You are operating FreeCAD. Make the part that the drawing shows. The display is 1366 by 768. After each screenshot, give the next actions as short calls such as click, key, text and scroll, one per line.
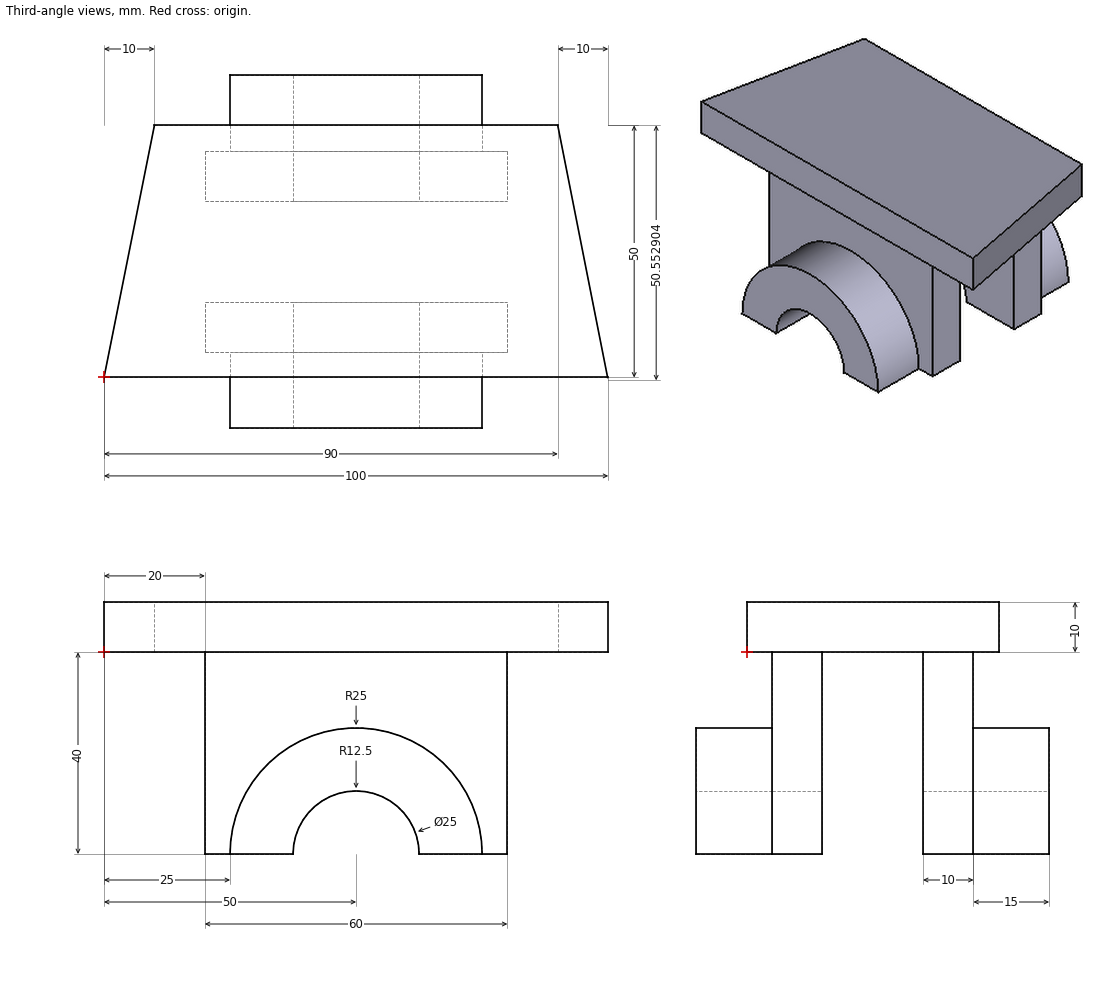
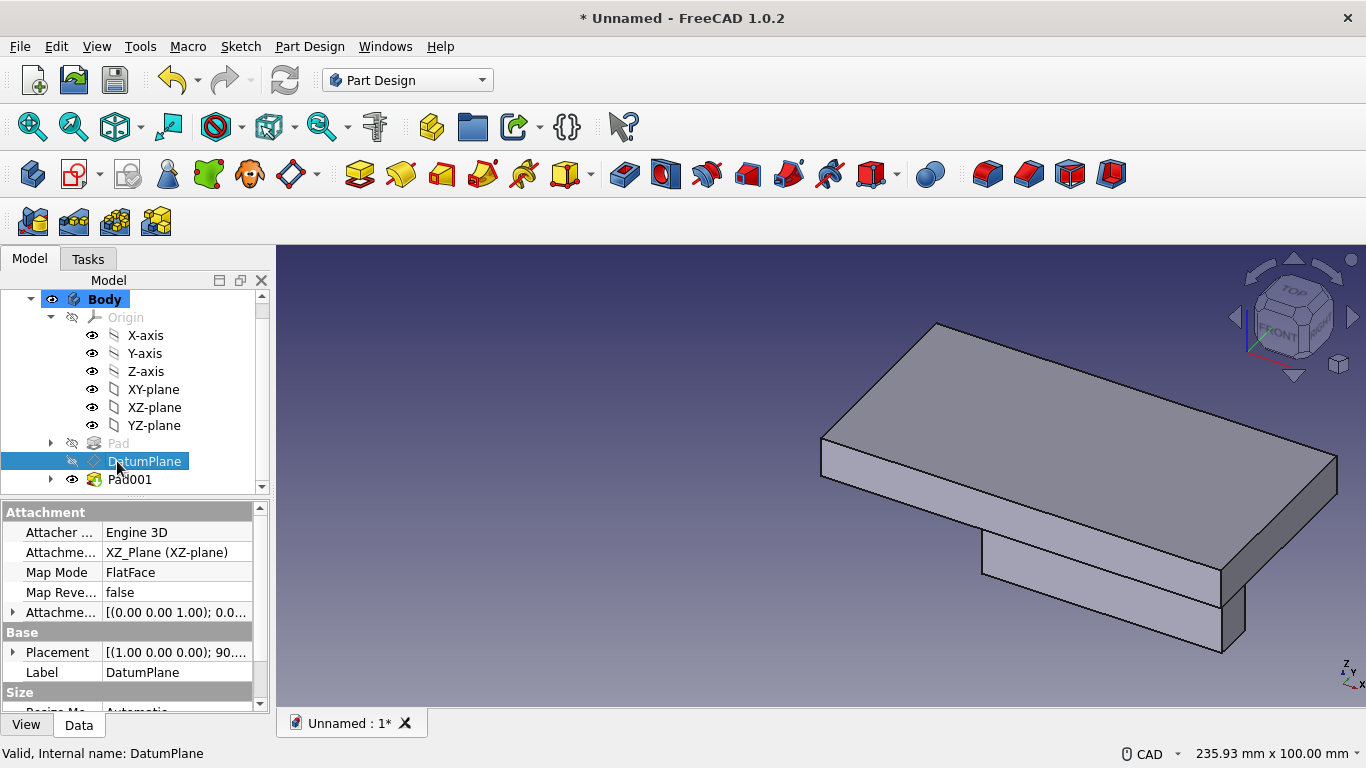
key(v)
key(f)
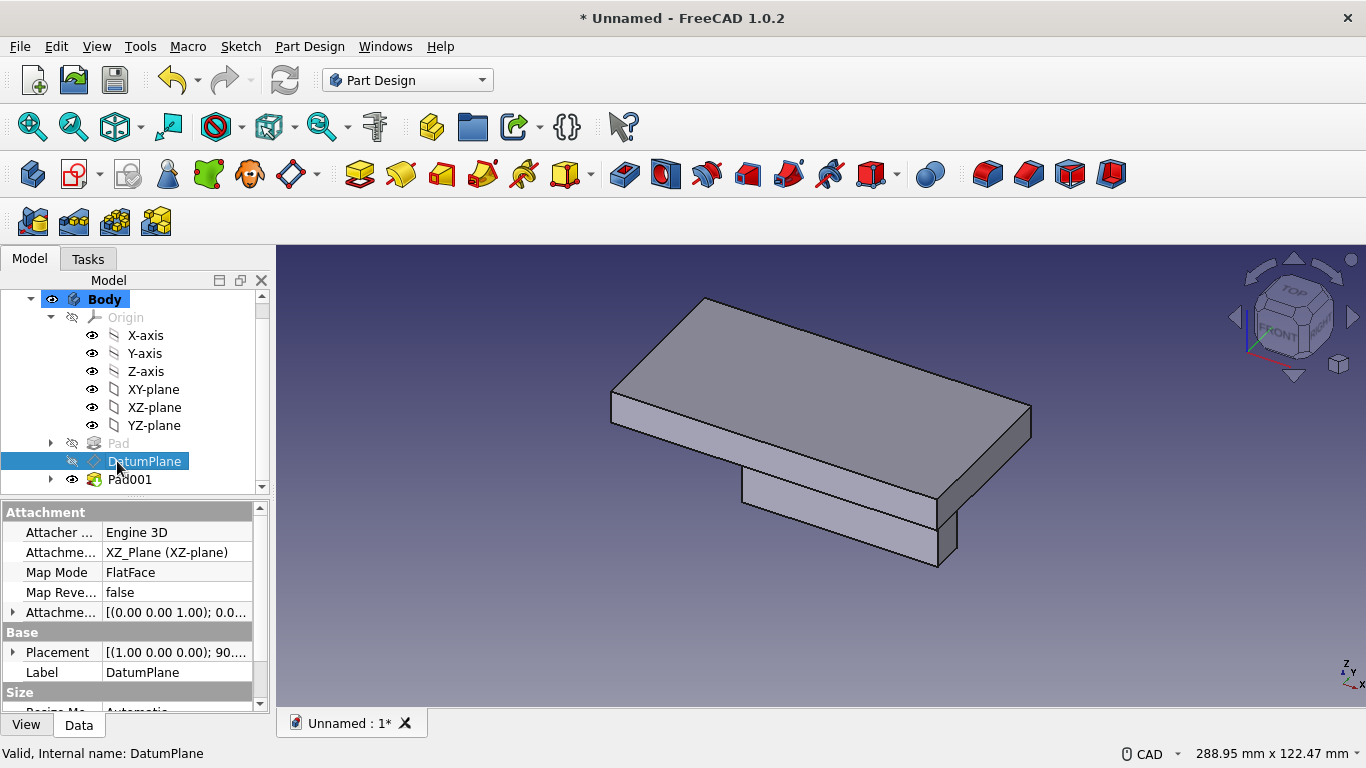
click(137, 407)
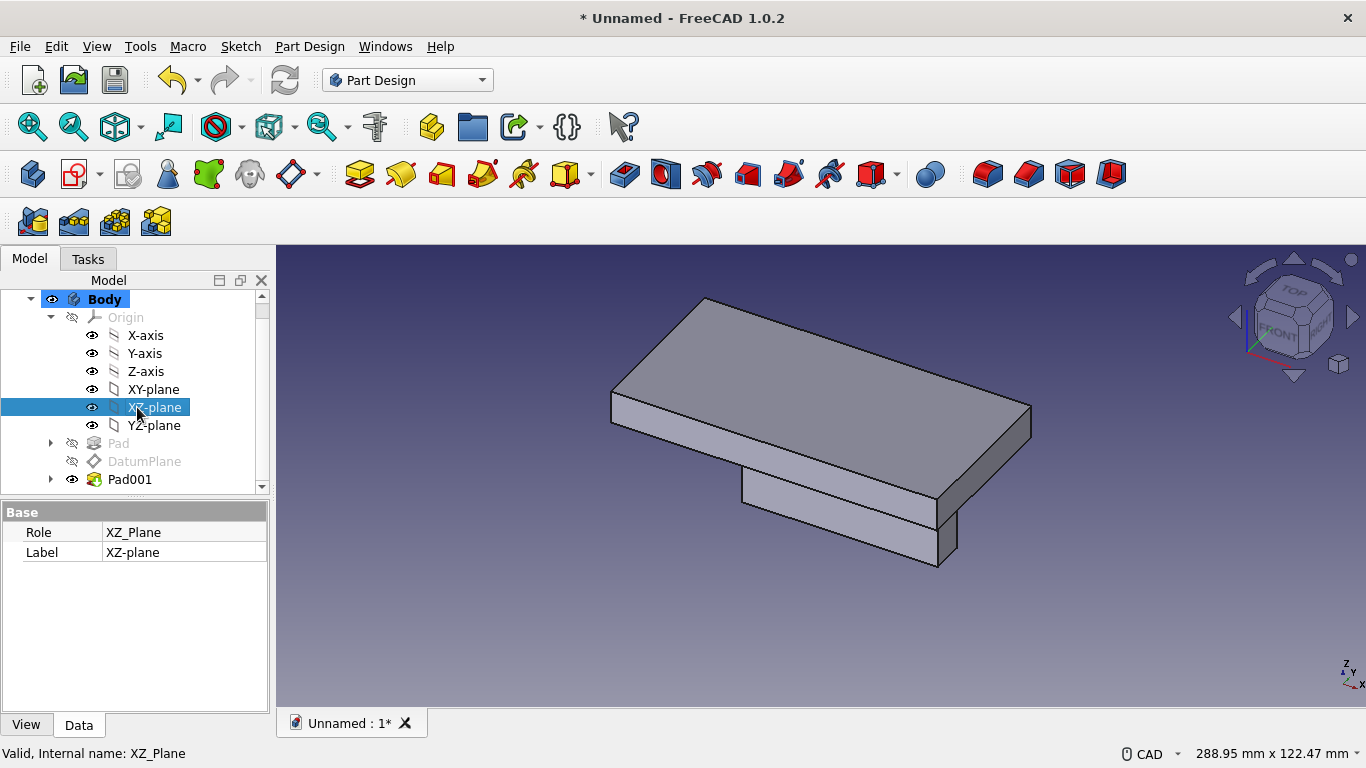
click(290, 174)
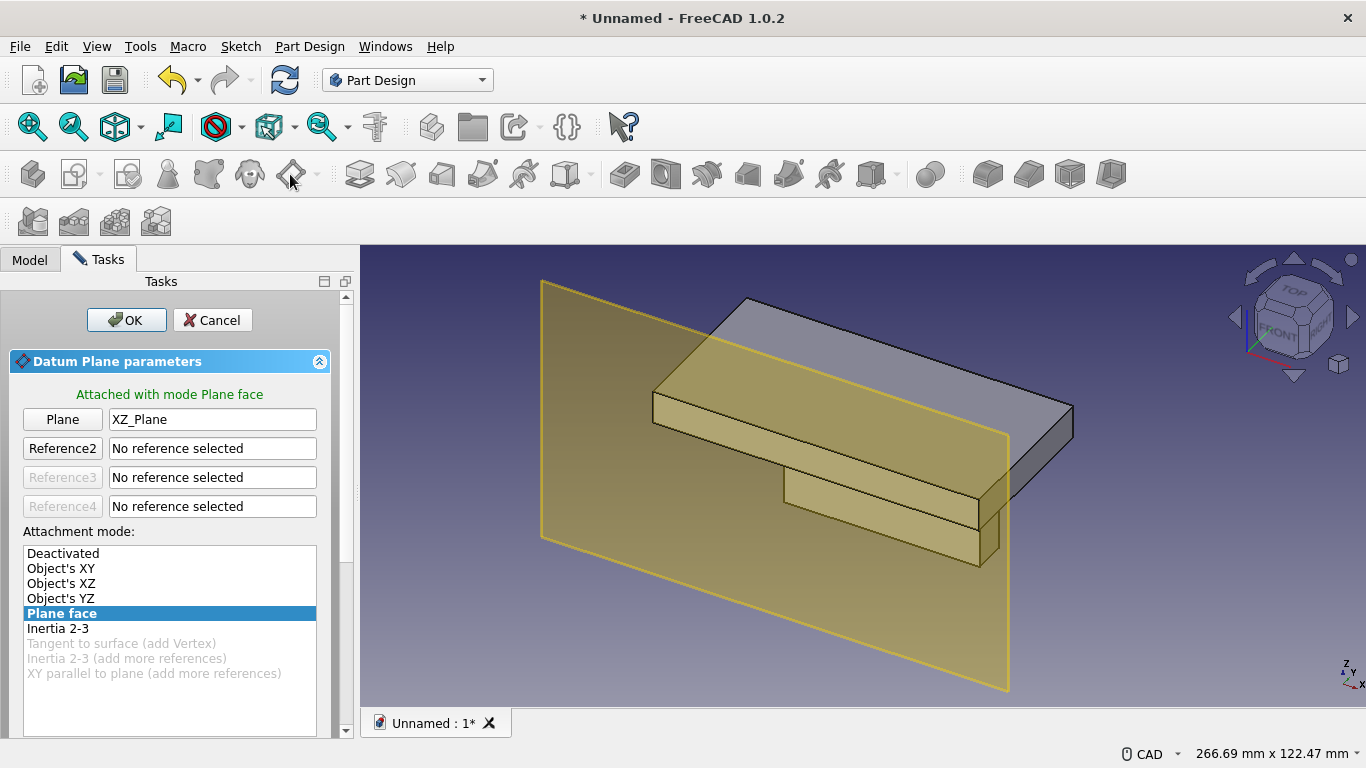
scroll(346, 514, down, 4)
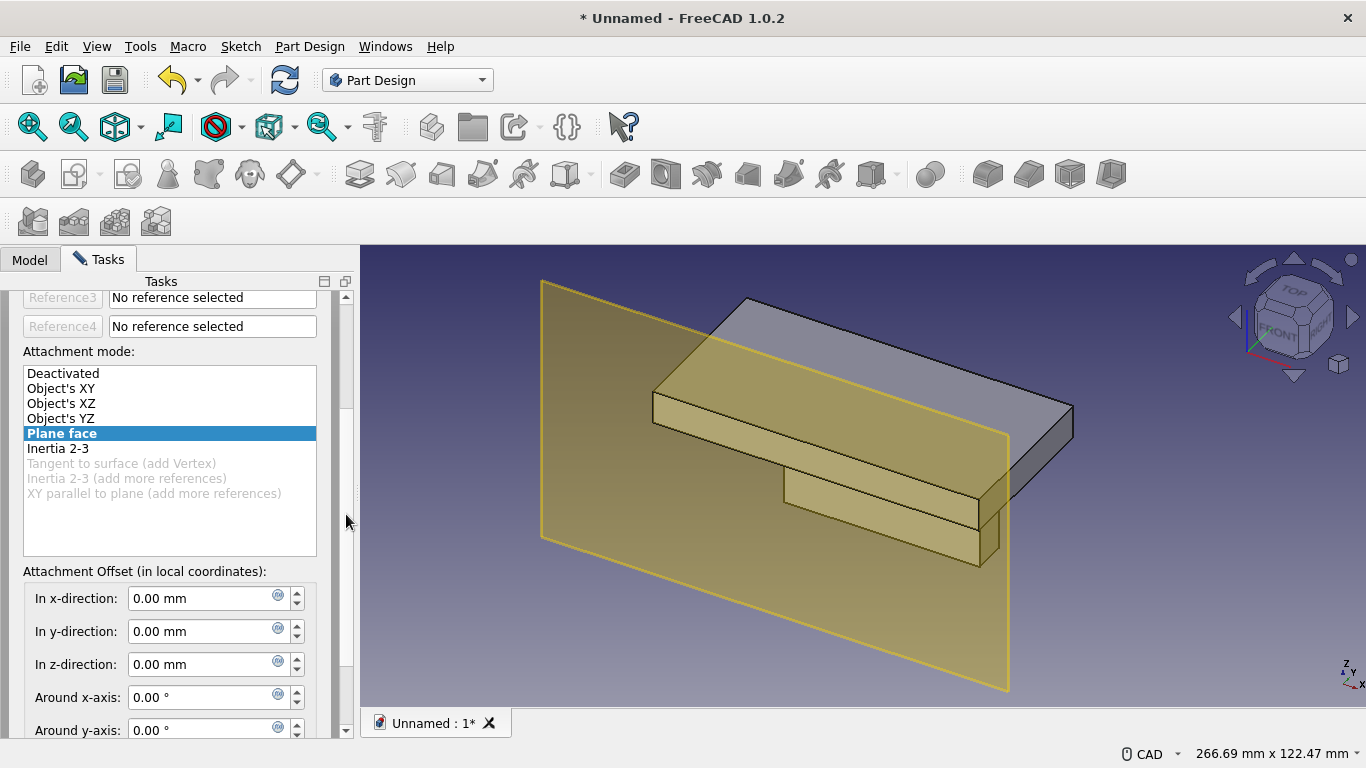
triple_click(210, 604)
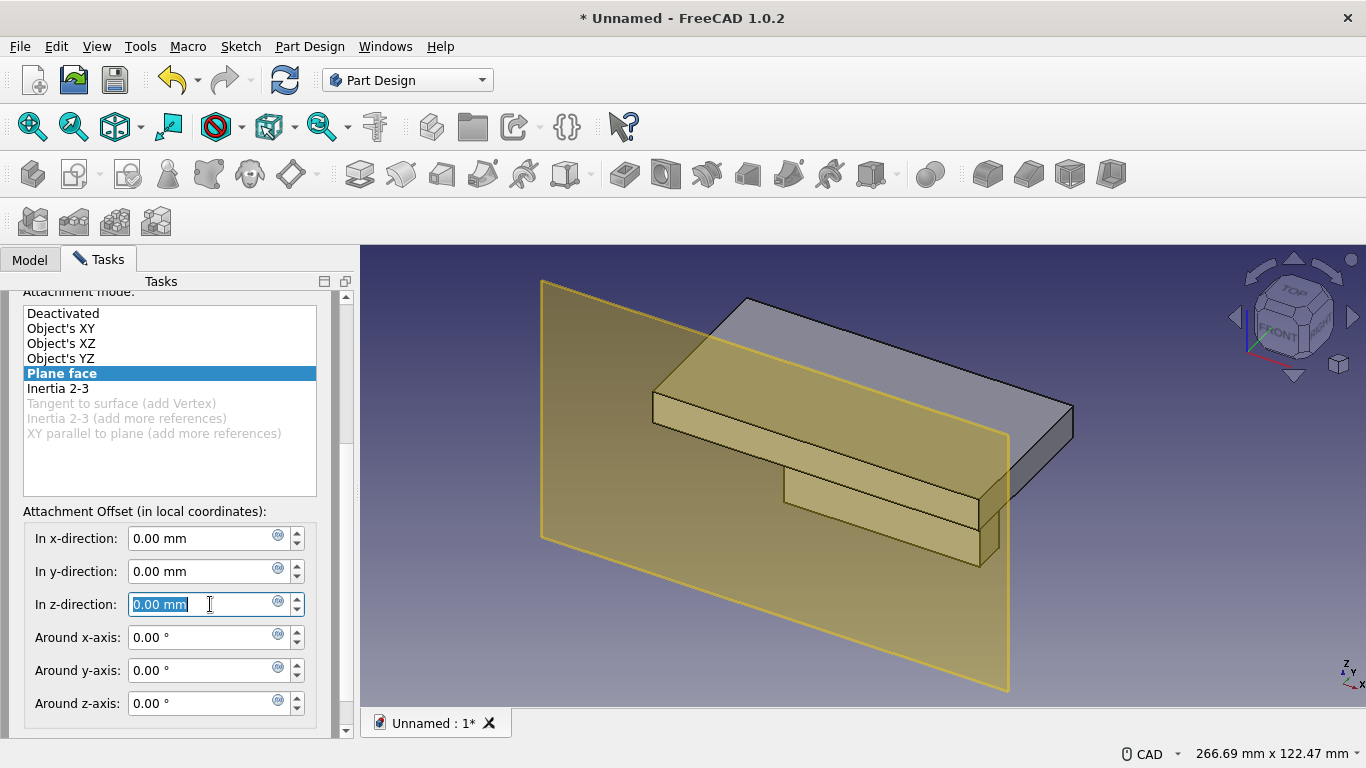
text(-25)
key(Tab)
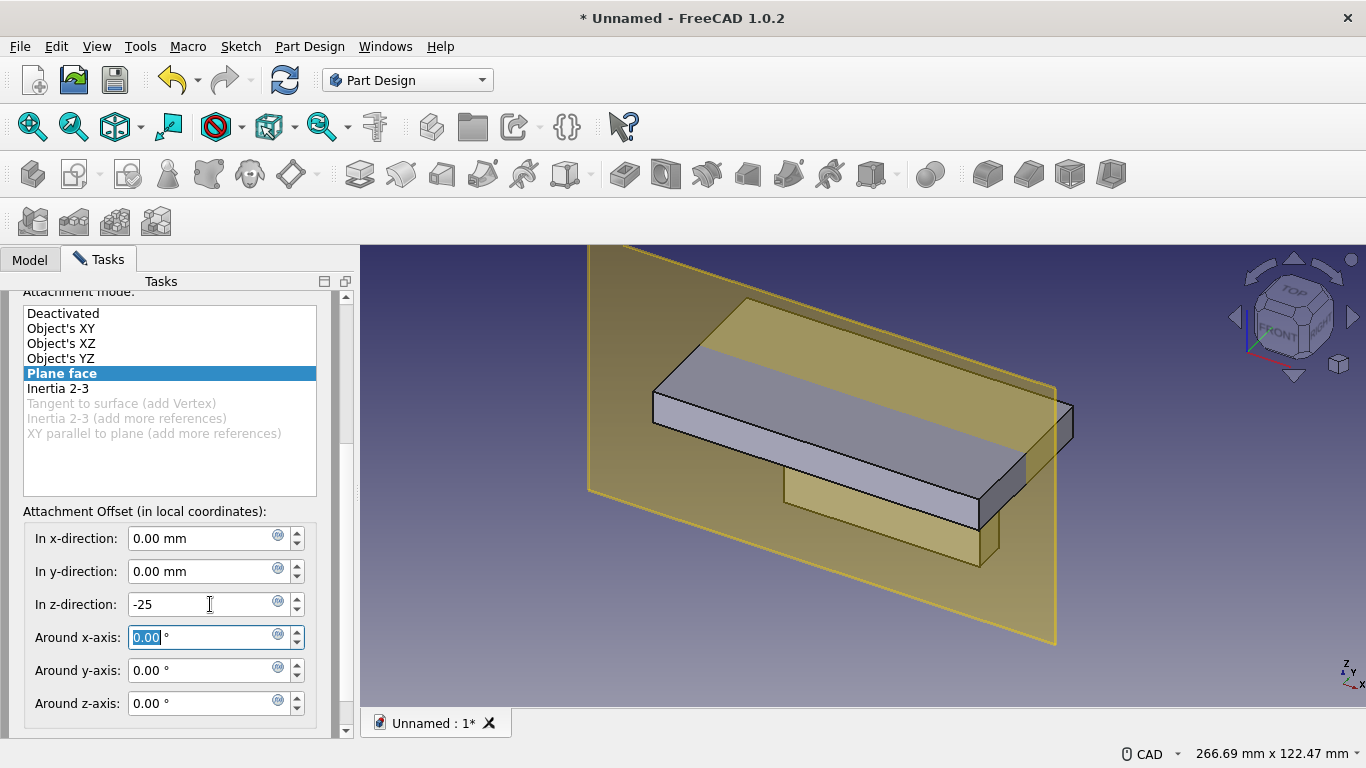
scroll(346, 514, up, 5)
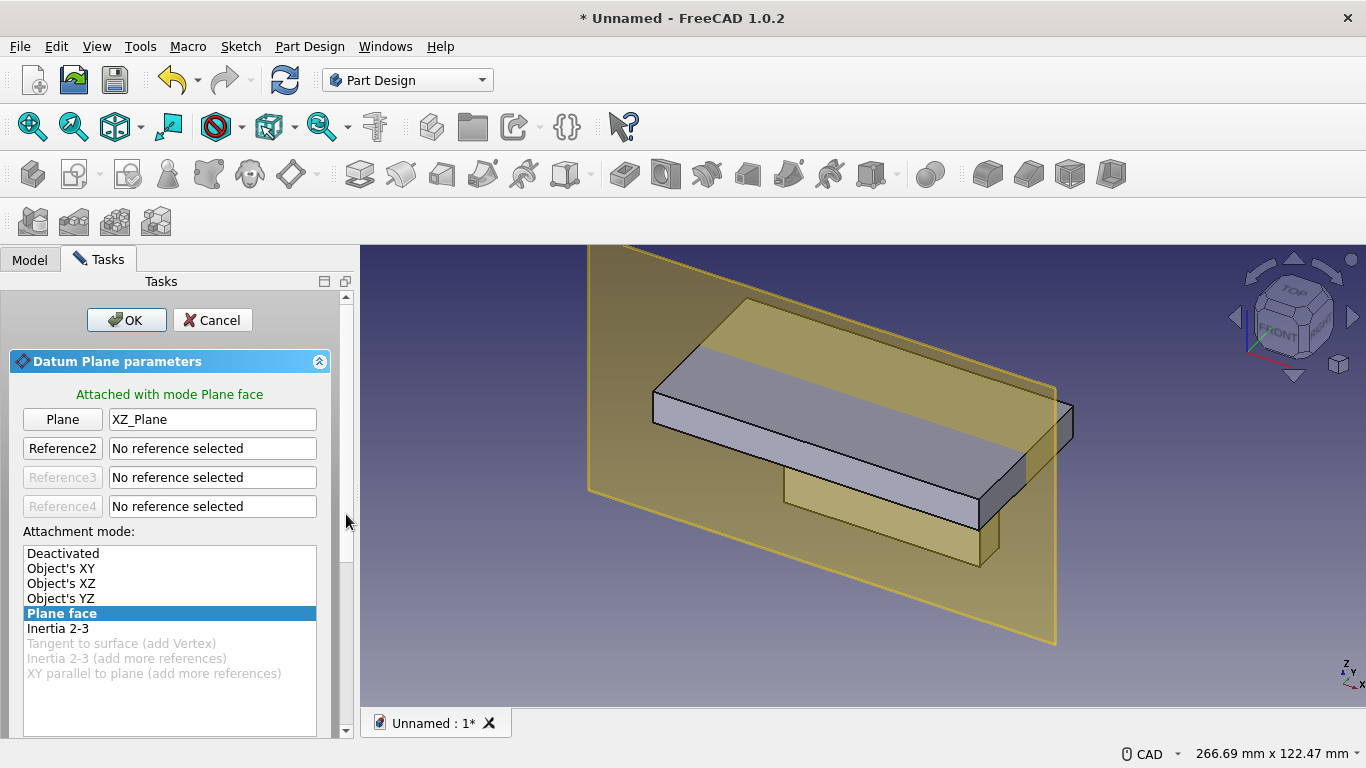
click(127, 320)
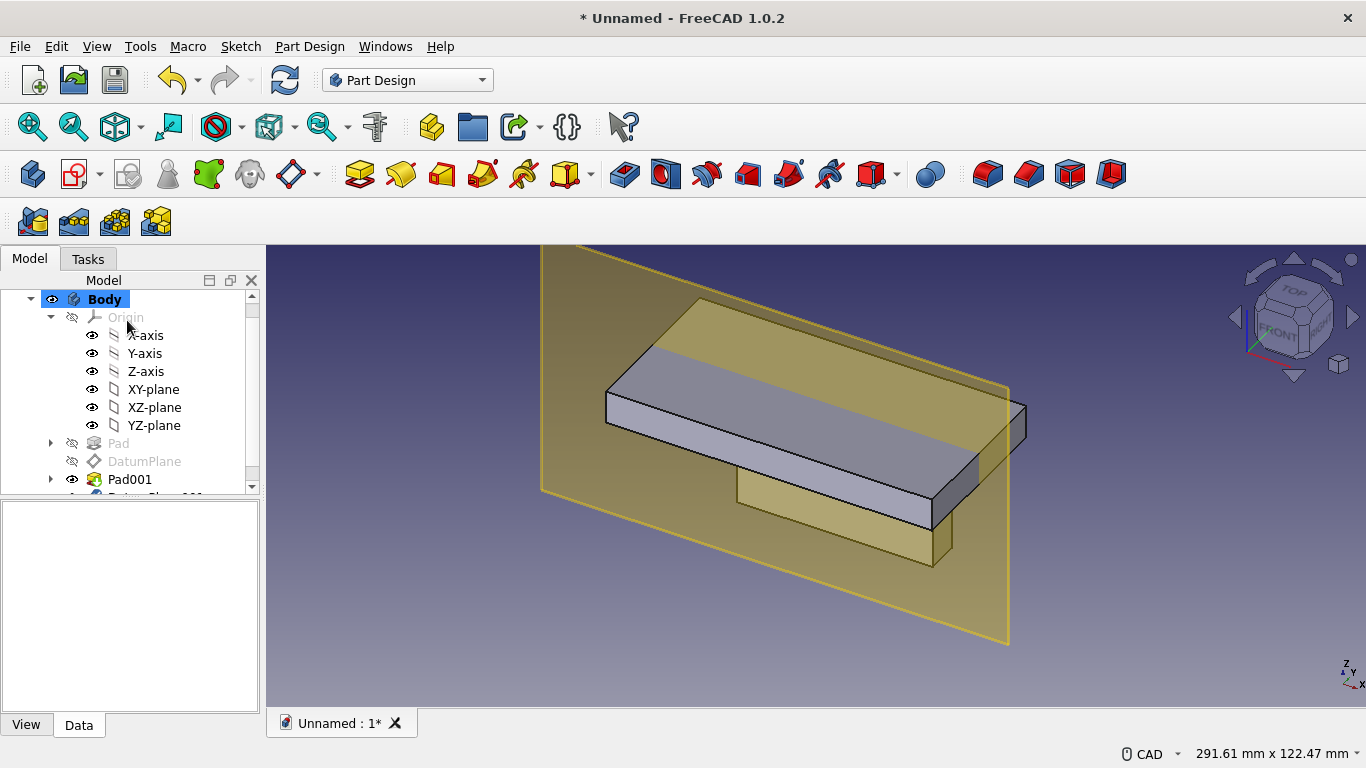
click(117, 479)